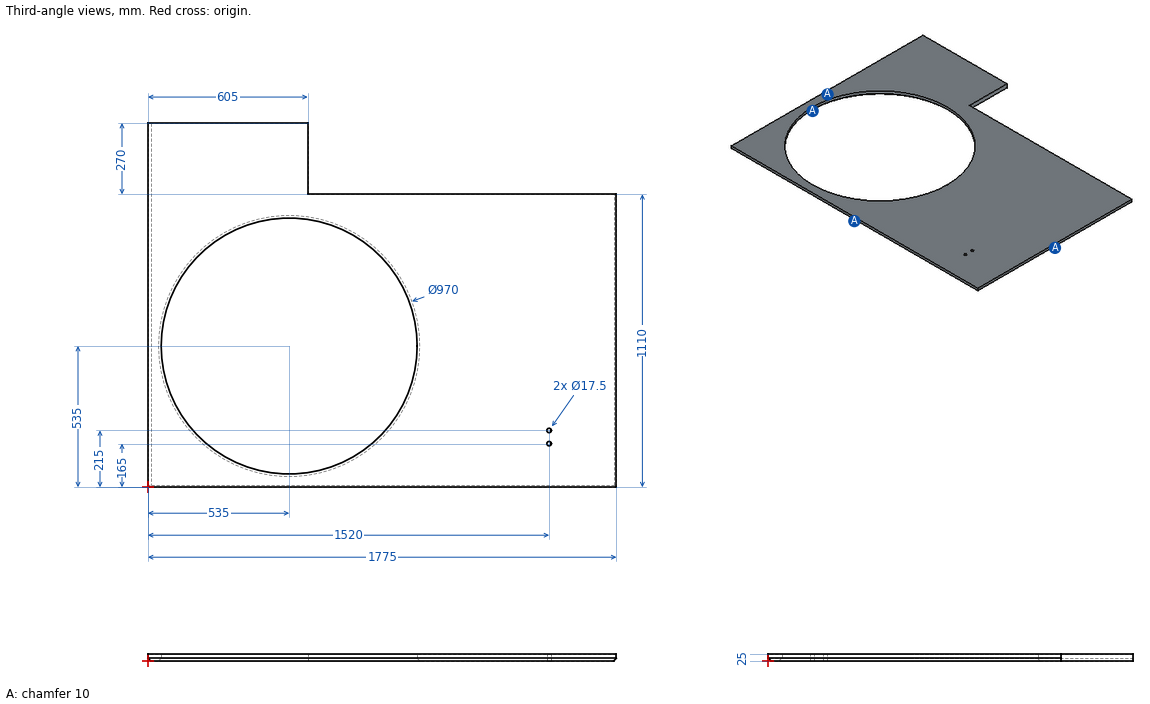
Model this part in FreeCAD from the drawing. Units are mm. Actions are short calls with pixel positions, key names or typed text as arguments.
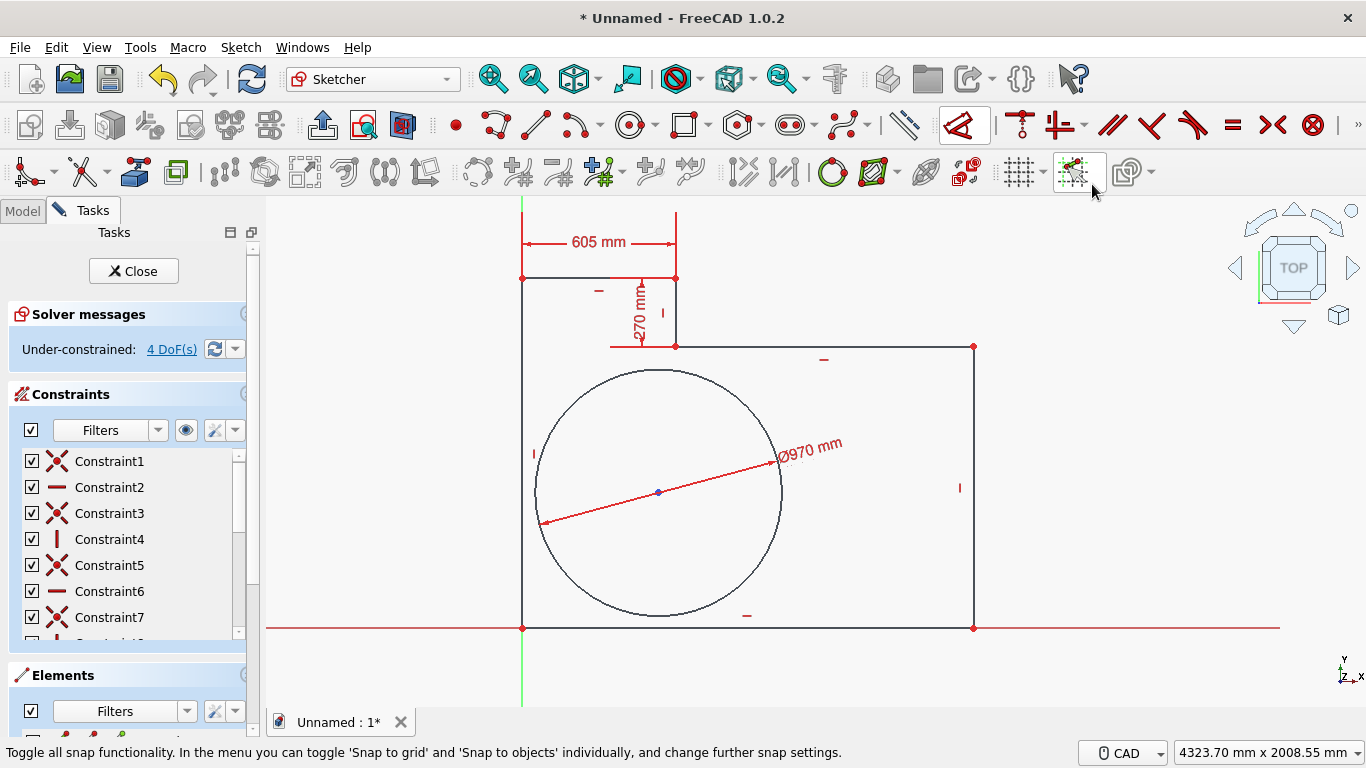
click(659, 493)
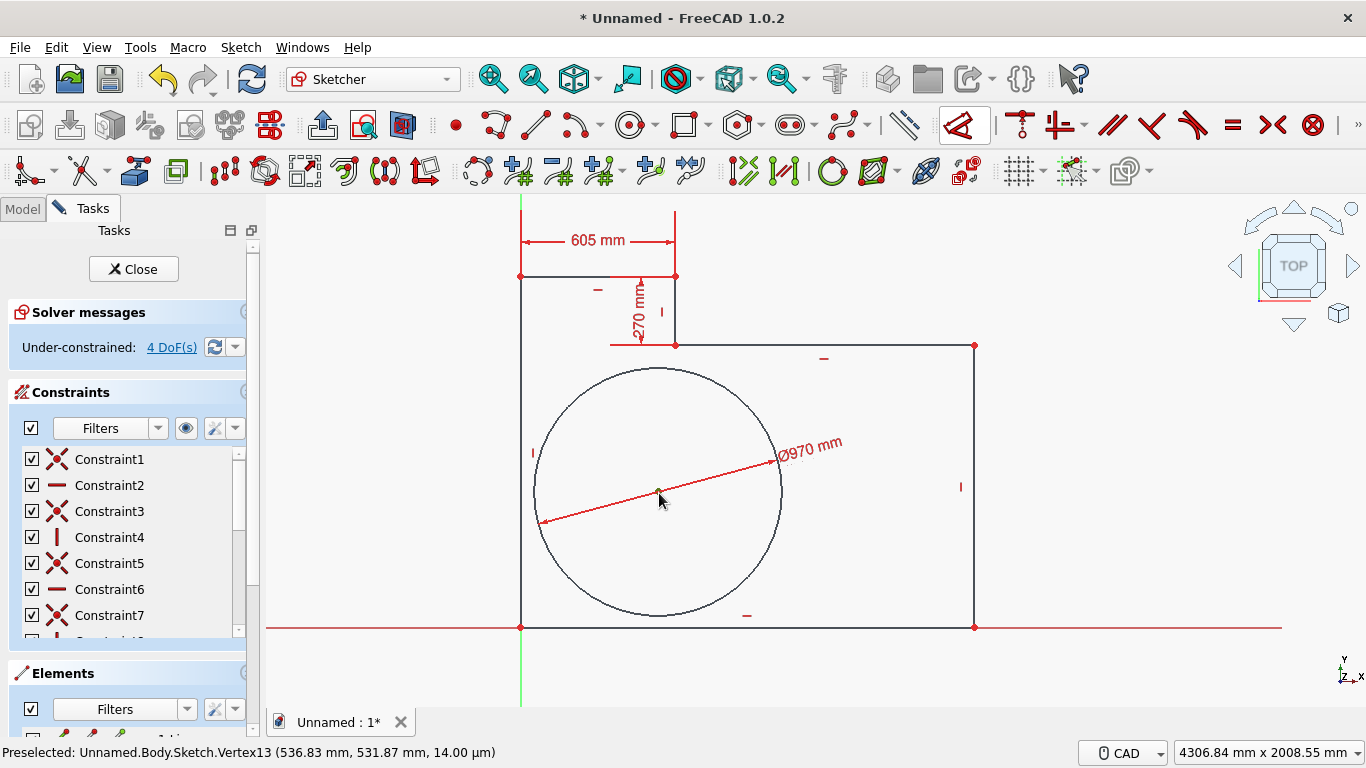
click(984, 126)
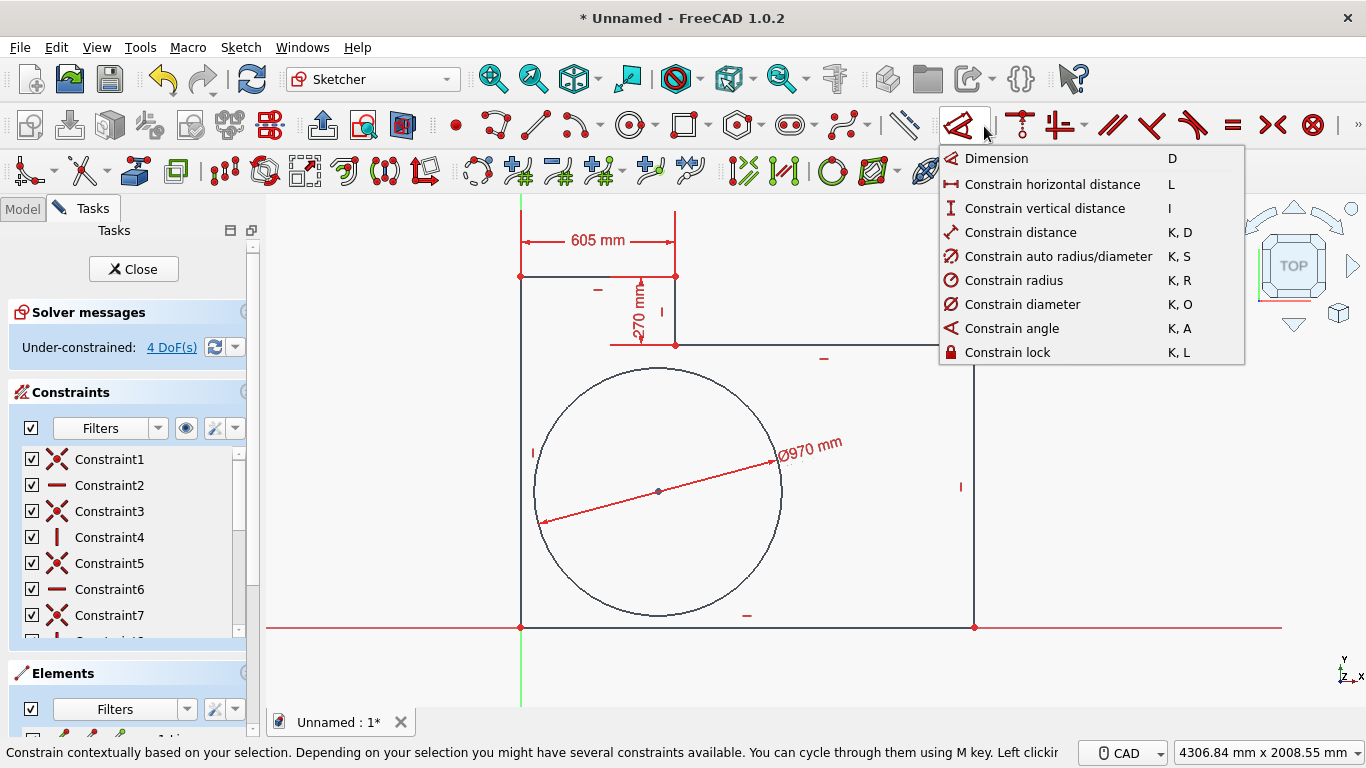
click(1092, 184)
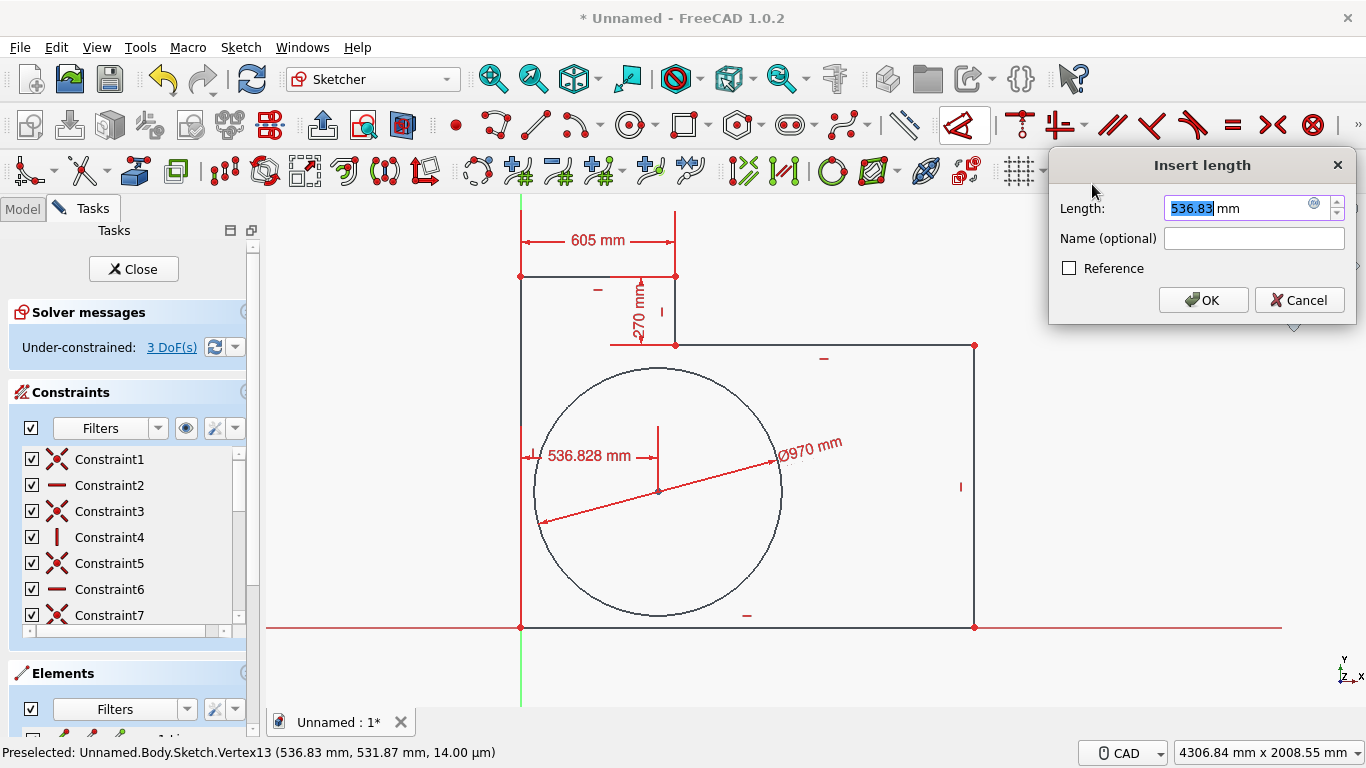
text(535)
key(Return)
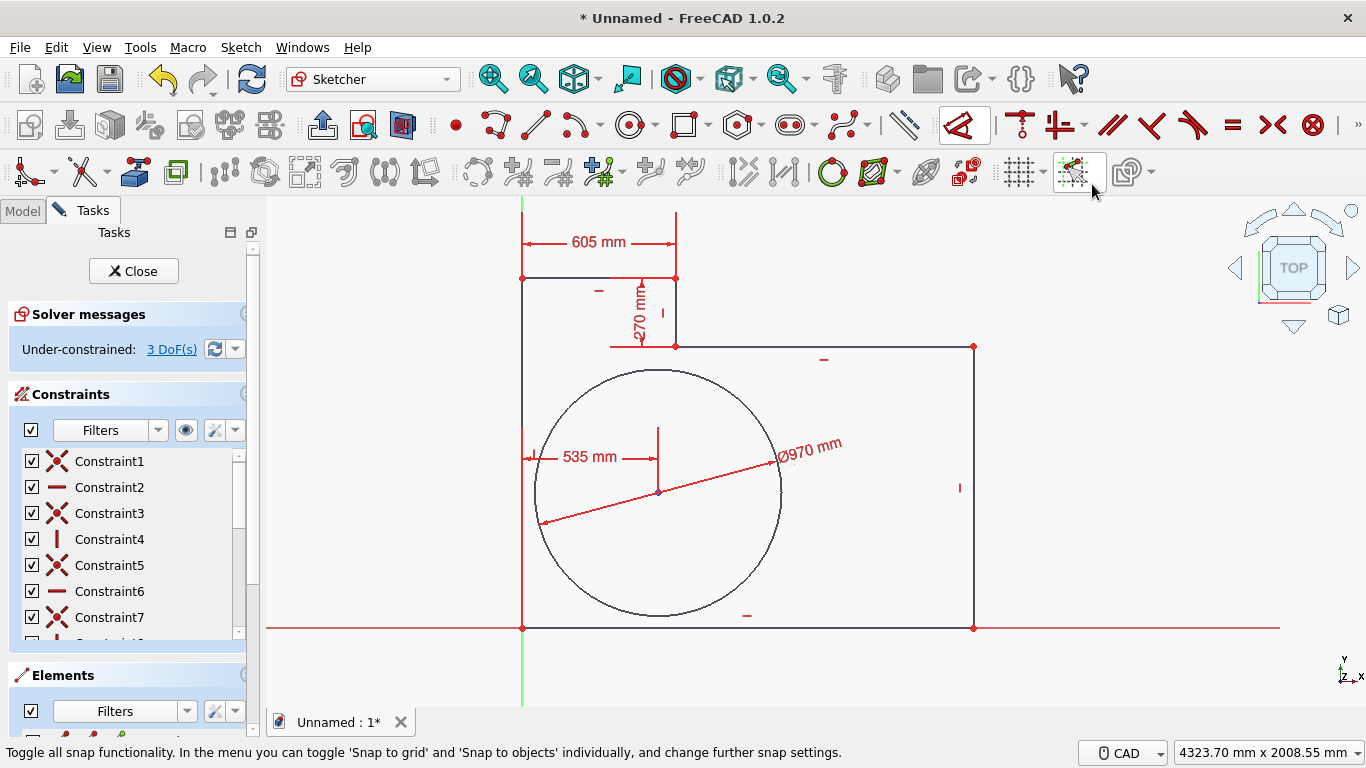
click(658, 493)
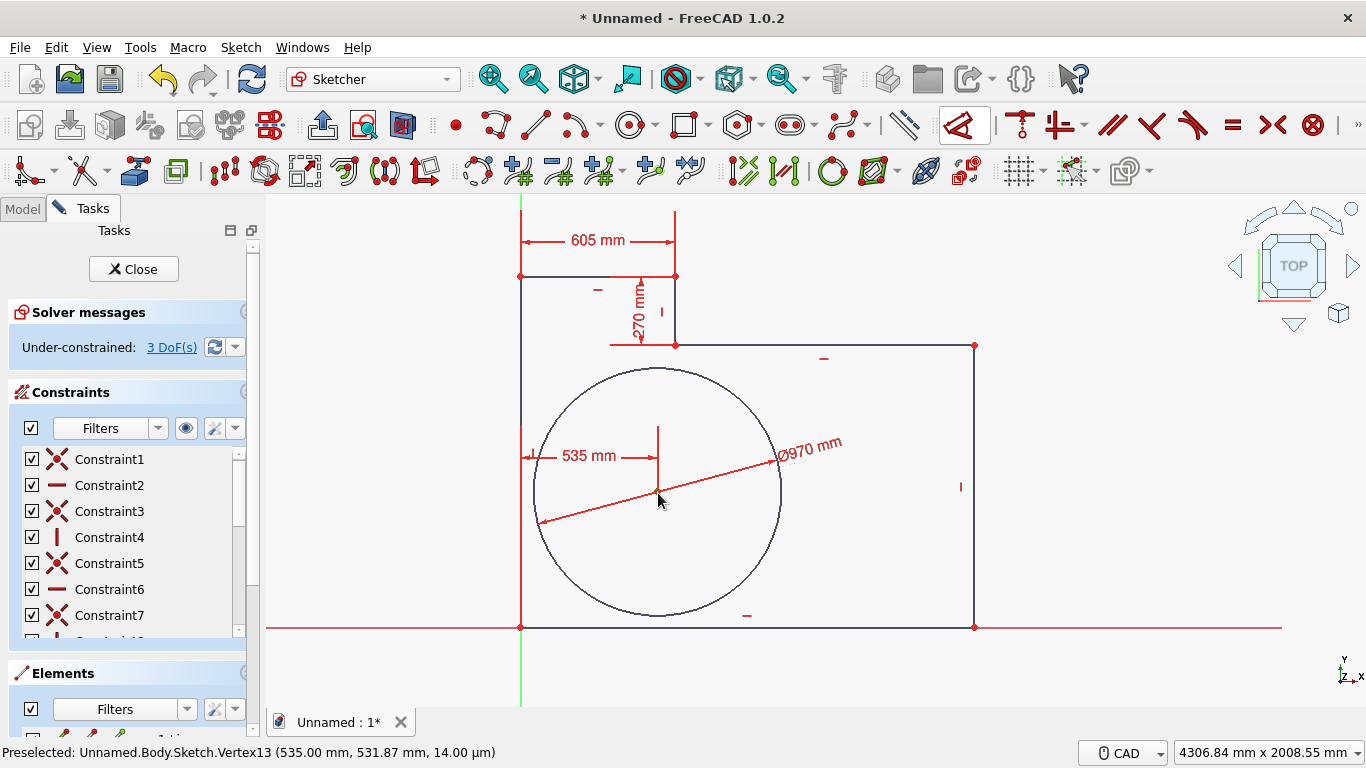
click(984, 126)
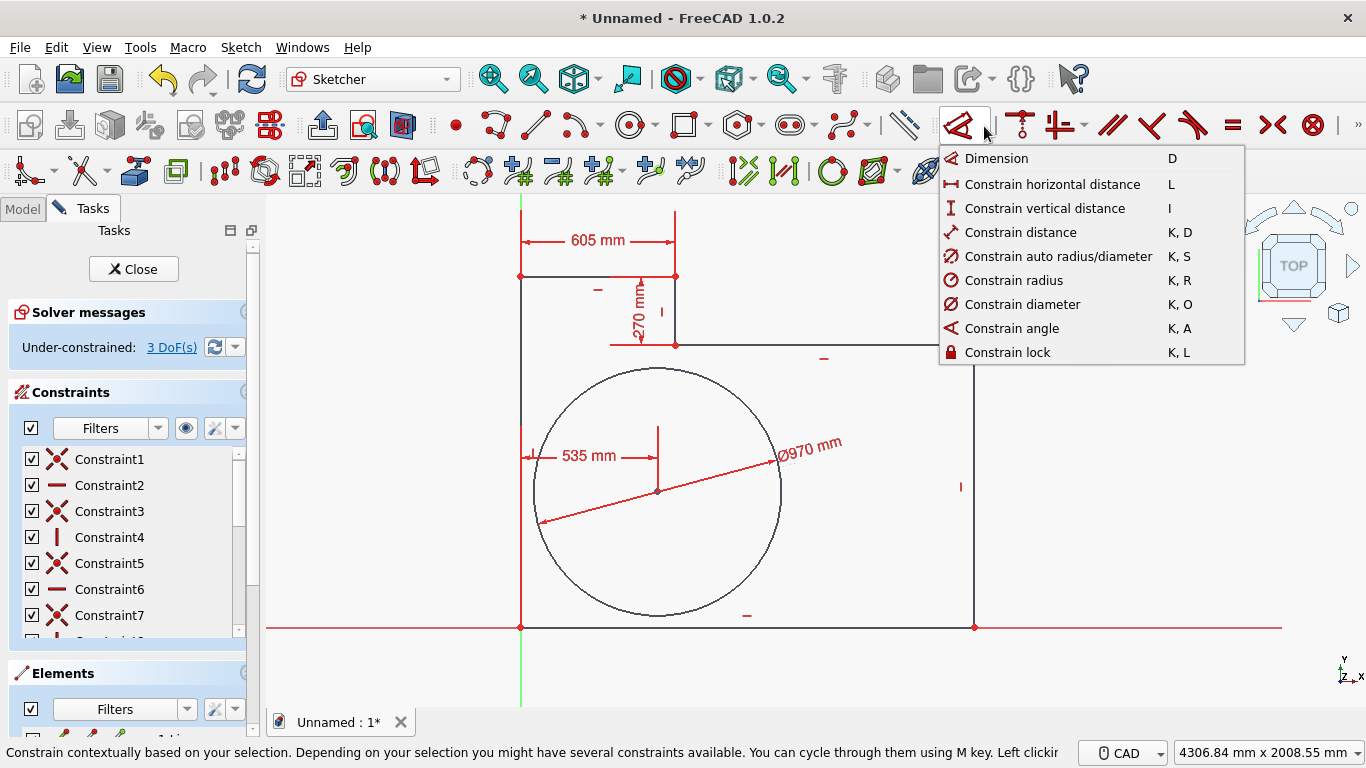
click(1092, 208)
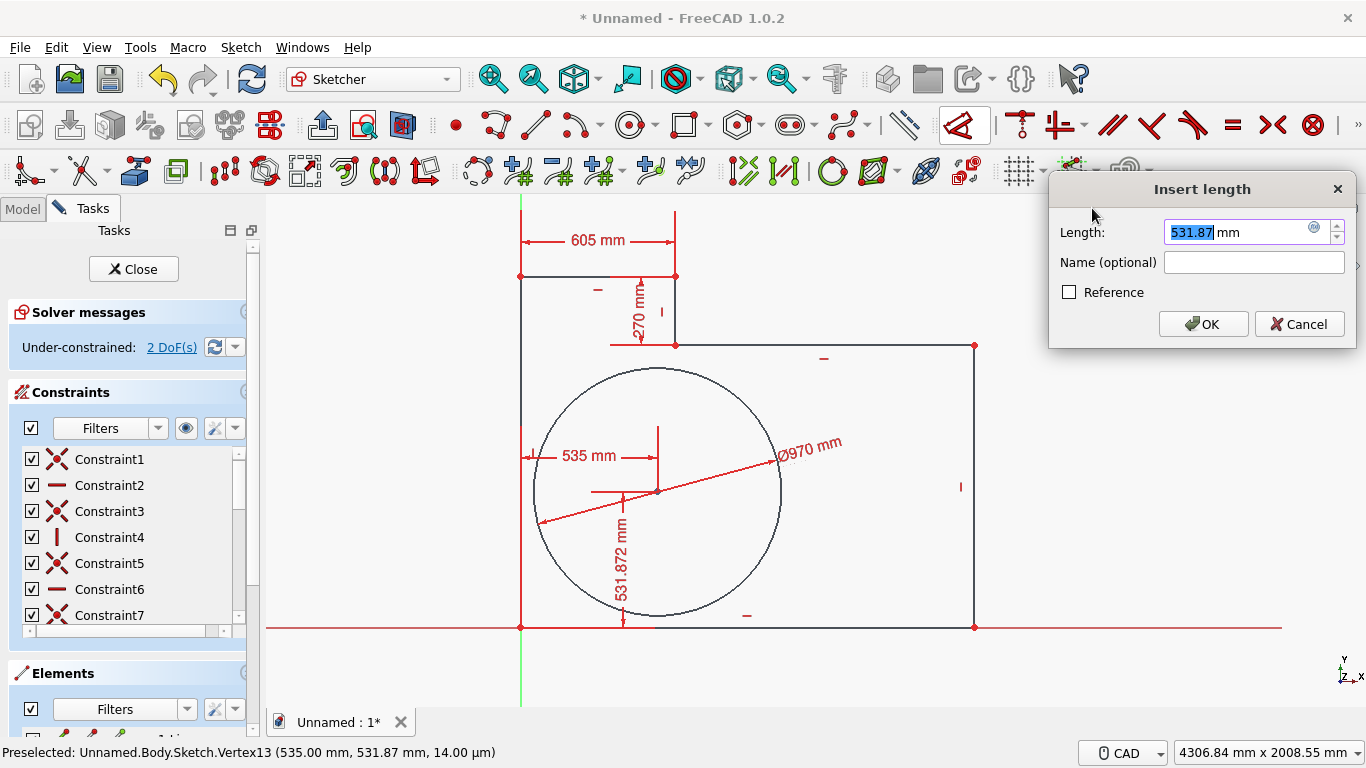
text(535)
key(Return)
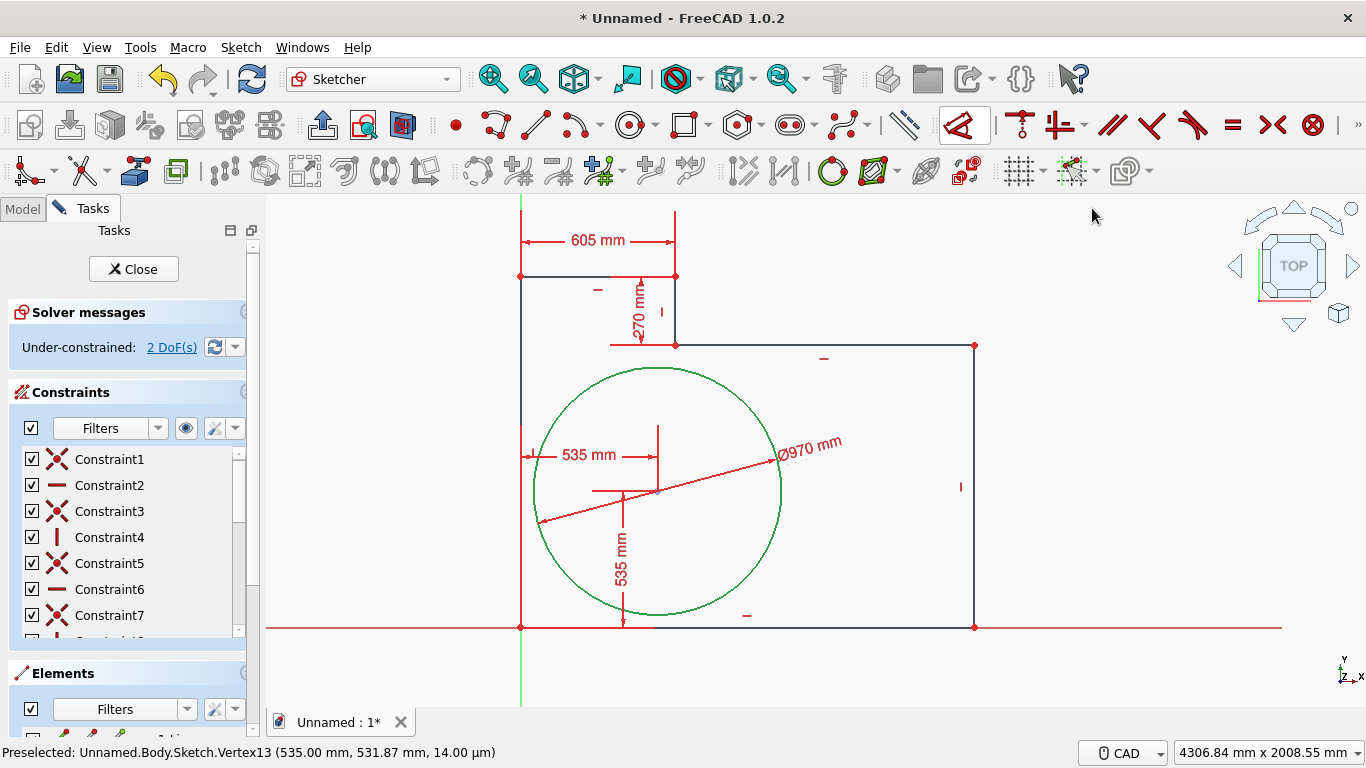
click(657, 628)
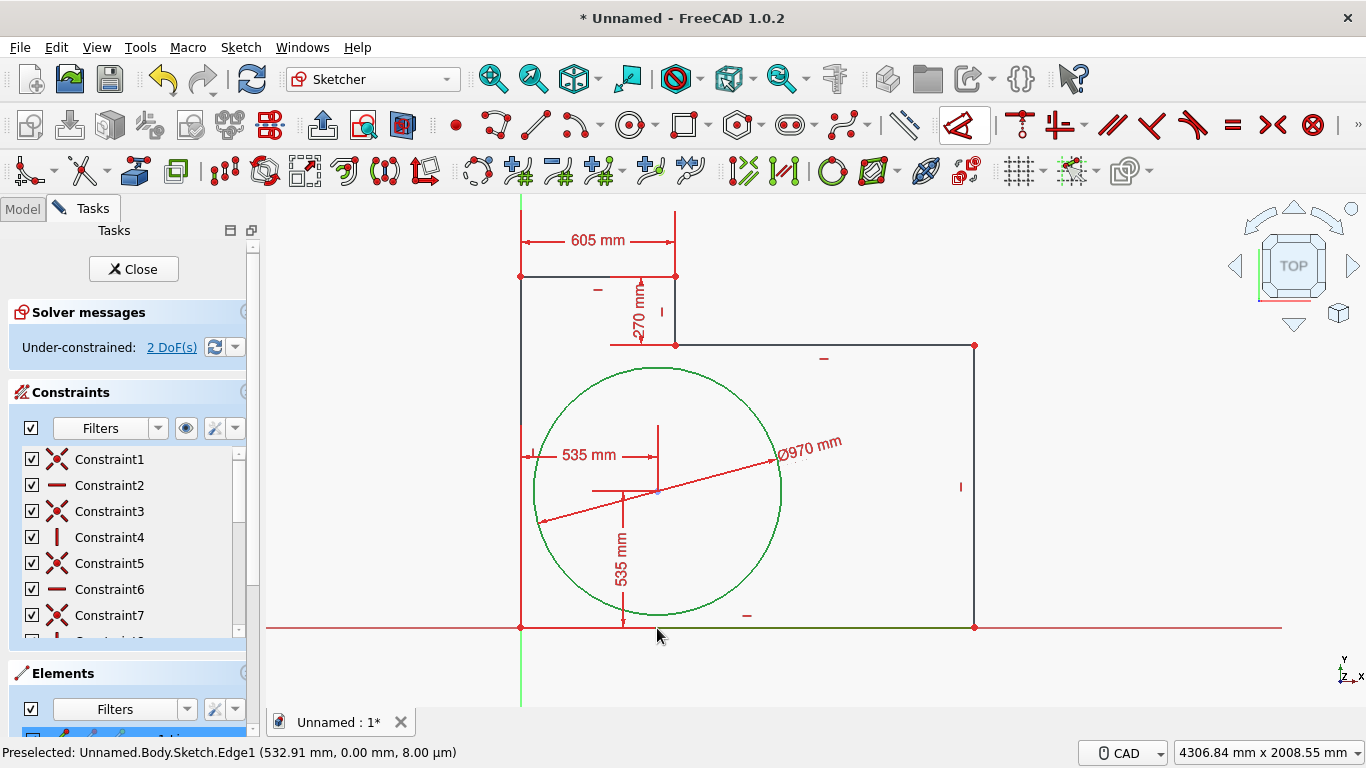
click(984, 126)